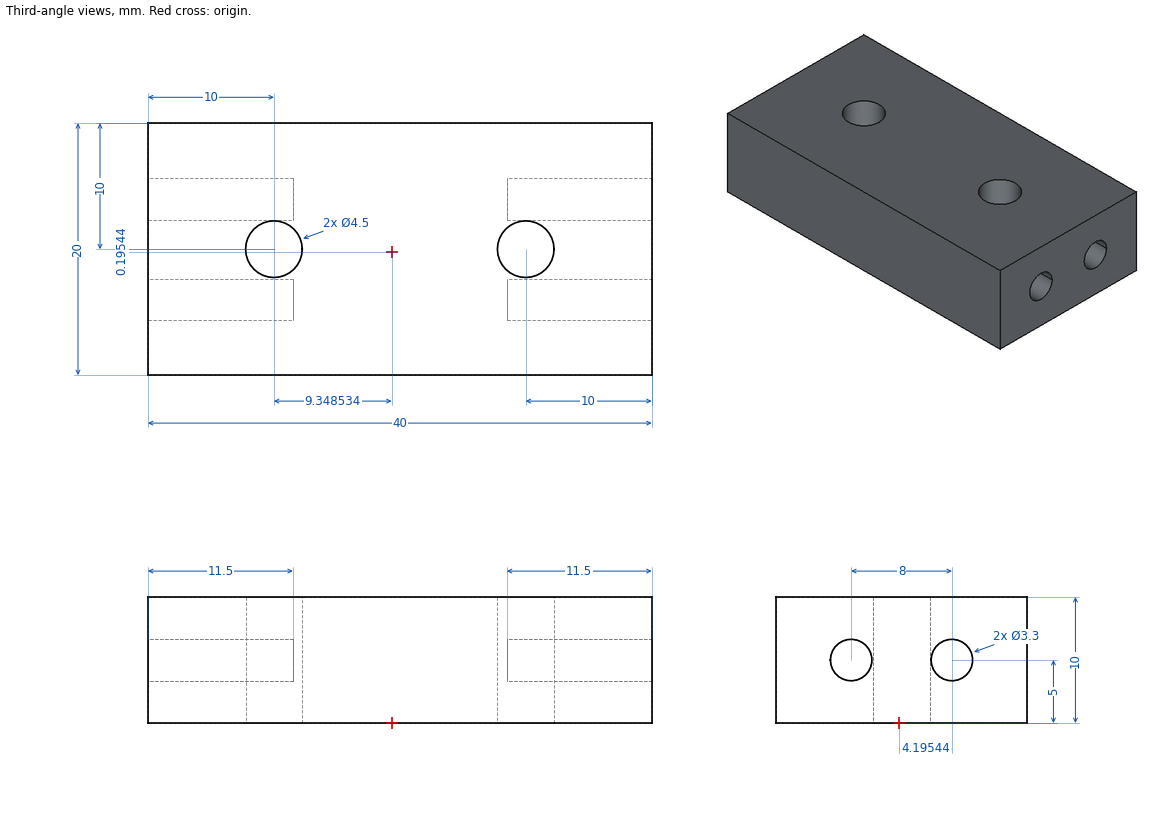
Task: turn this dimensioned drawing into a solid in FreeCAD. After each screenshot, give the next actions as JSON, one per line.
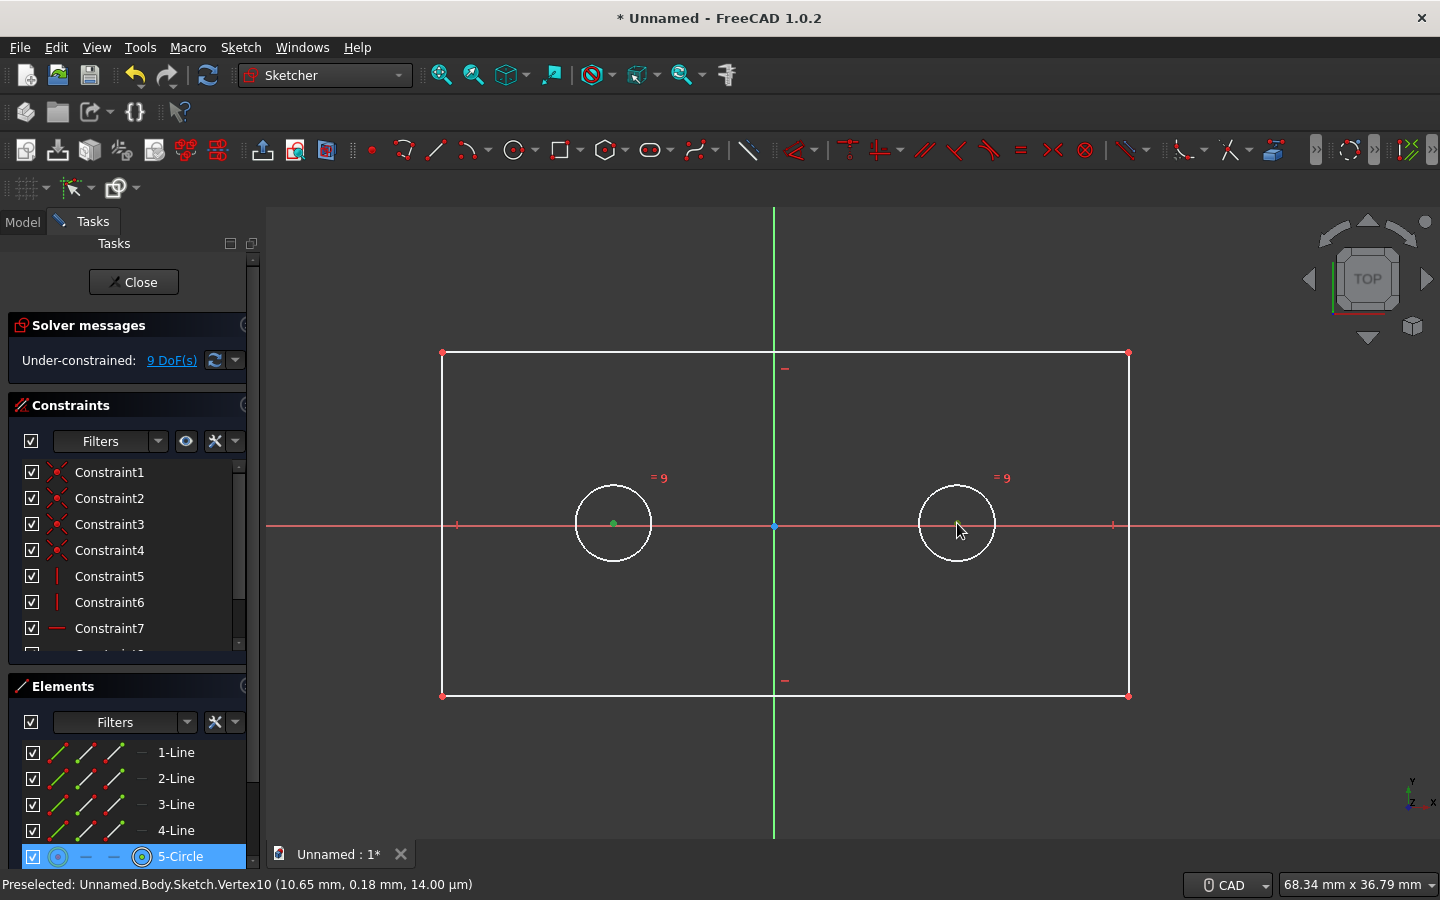
{"action": "key", "text": "h"}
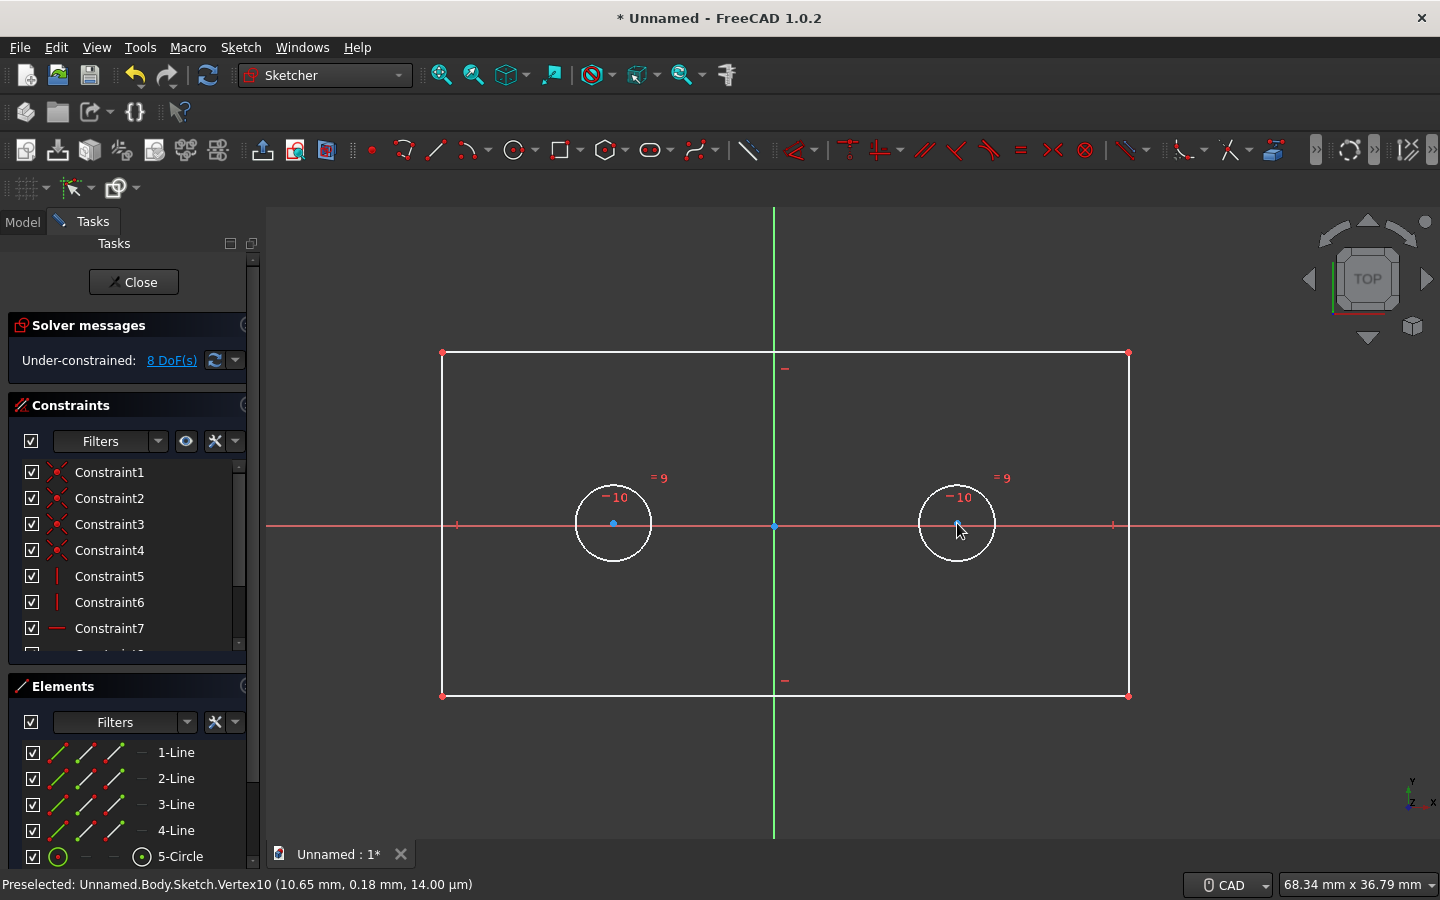
{"action": "key", "text": "d"}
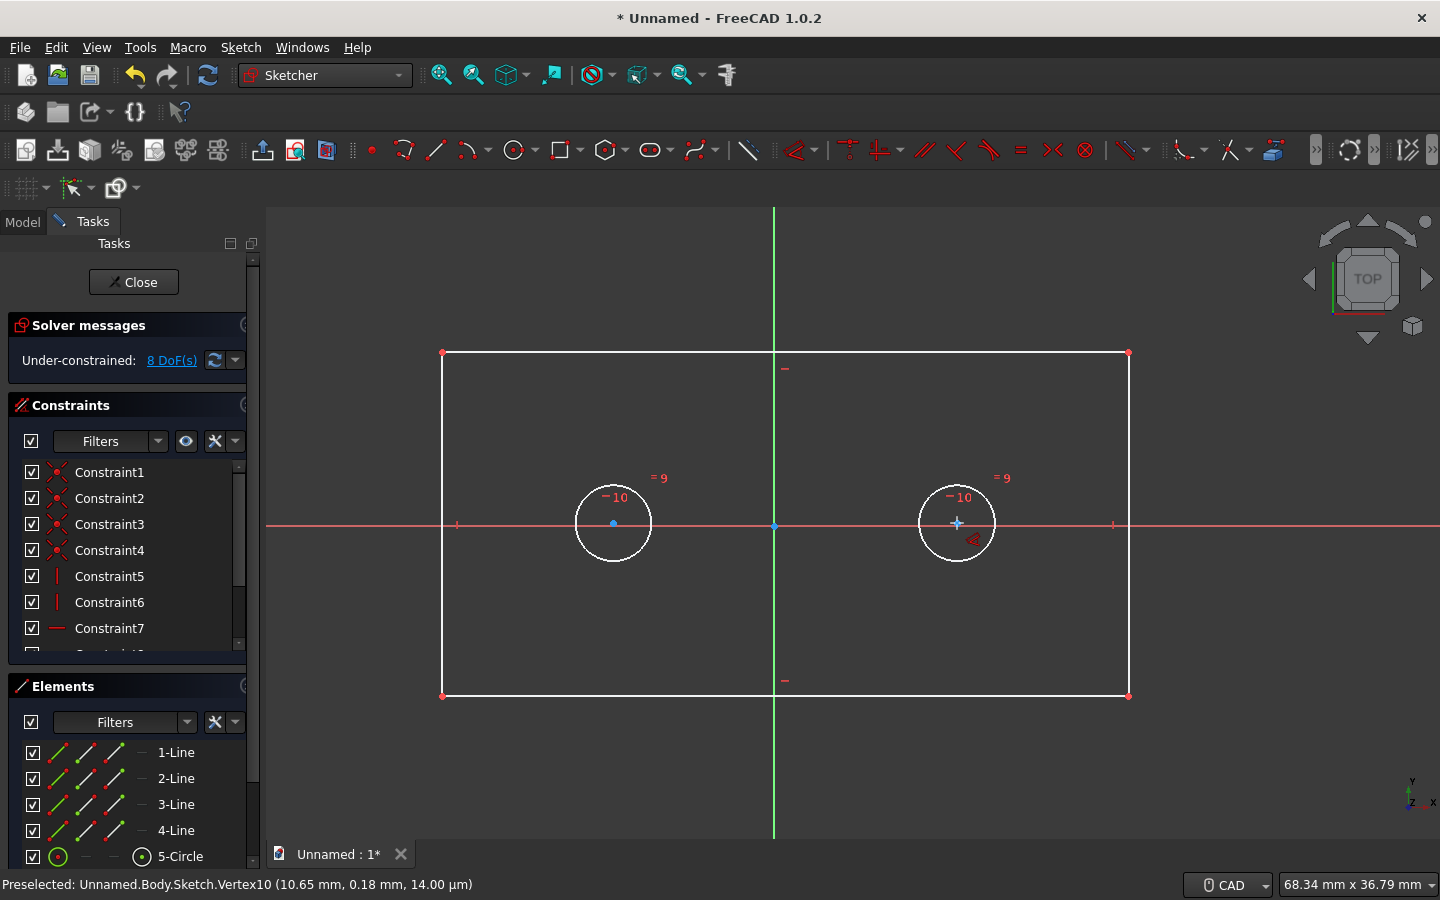
{"action": "left_click", "coordinate": [640, 496]}
{"action": "left_click", "coordinate": [662, 473]}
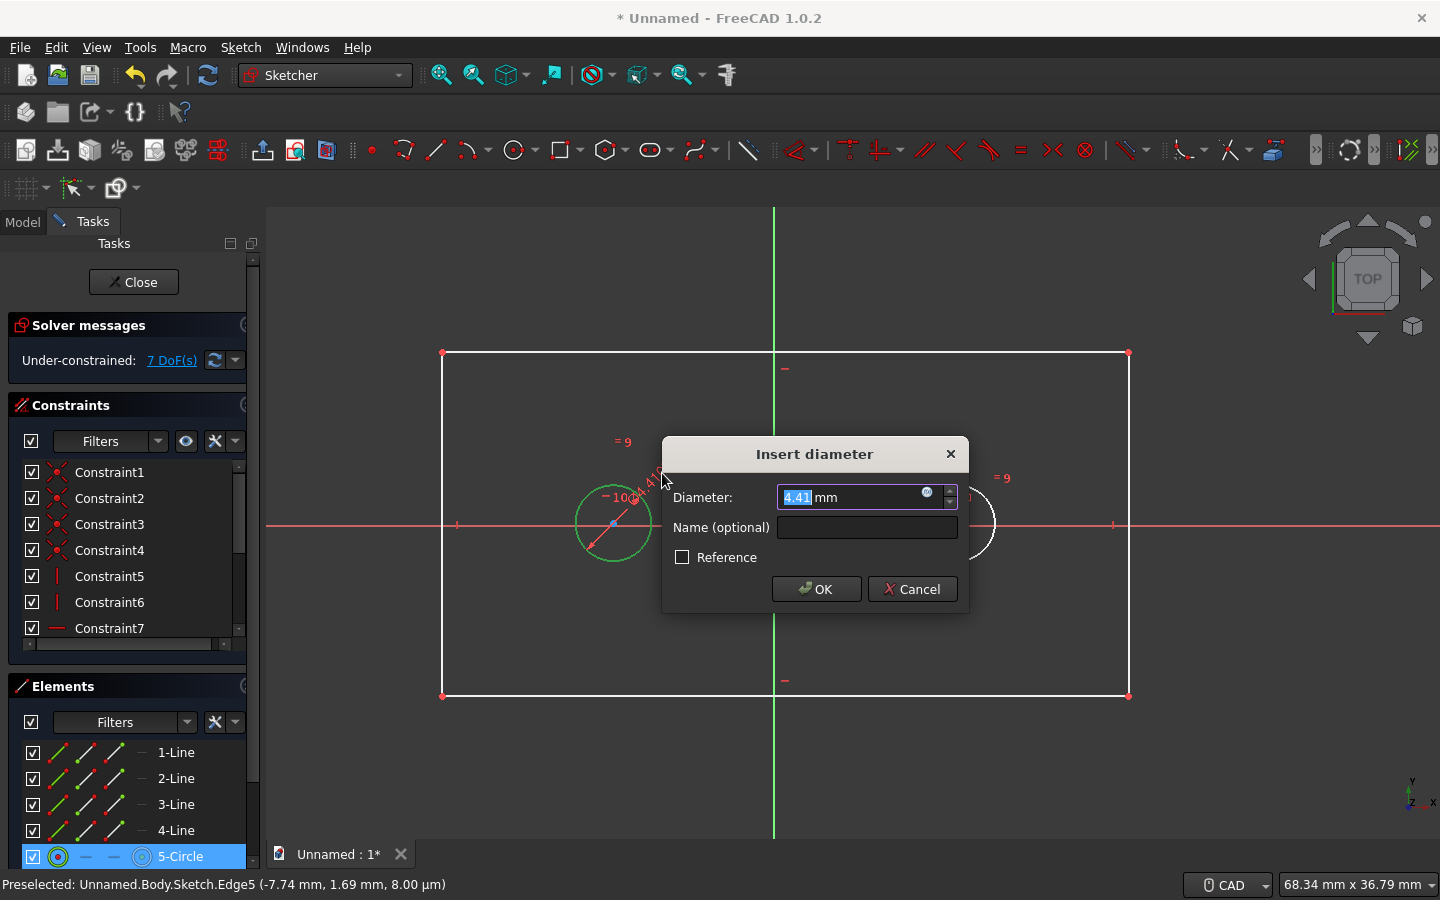
{"action": "type", "text": "4.5"}
{"action": "key", "text": "Return"}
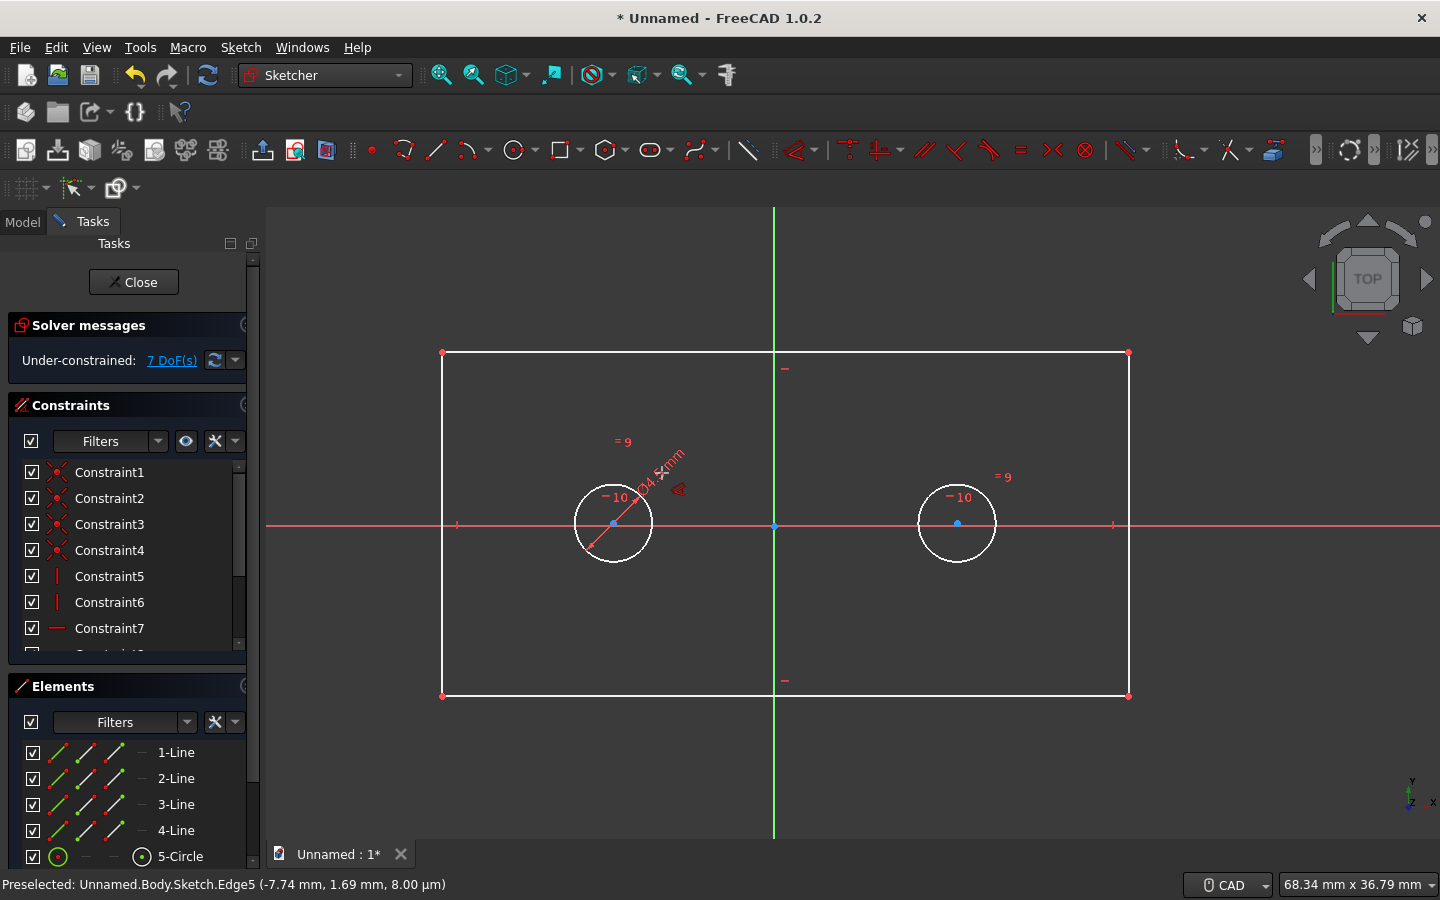
{"action": "left_click", "coordinate": [442, 456]}
{"action": "left_click", "coordinate": [408, 445]}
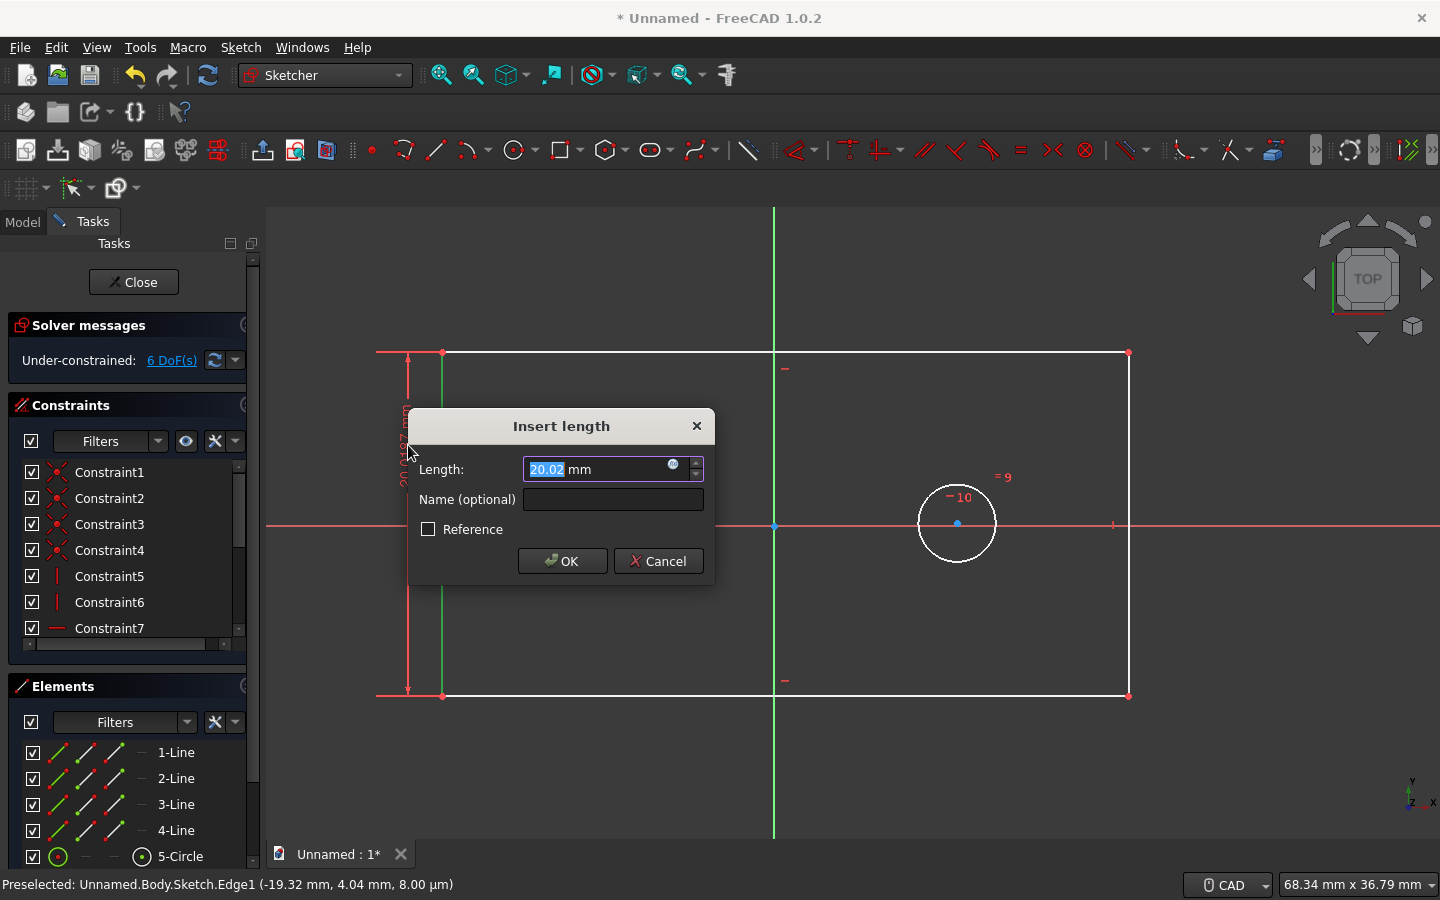
{"action": "type", "text": "20"}
{"action": "key", "text": "Return"}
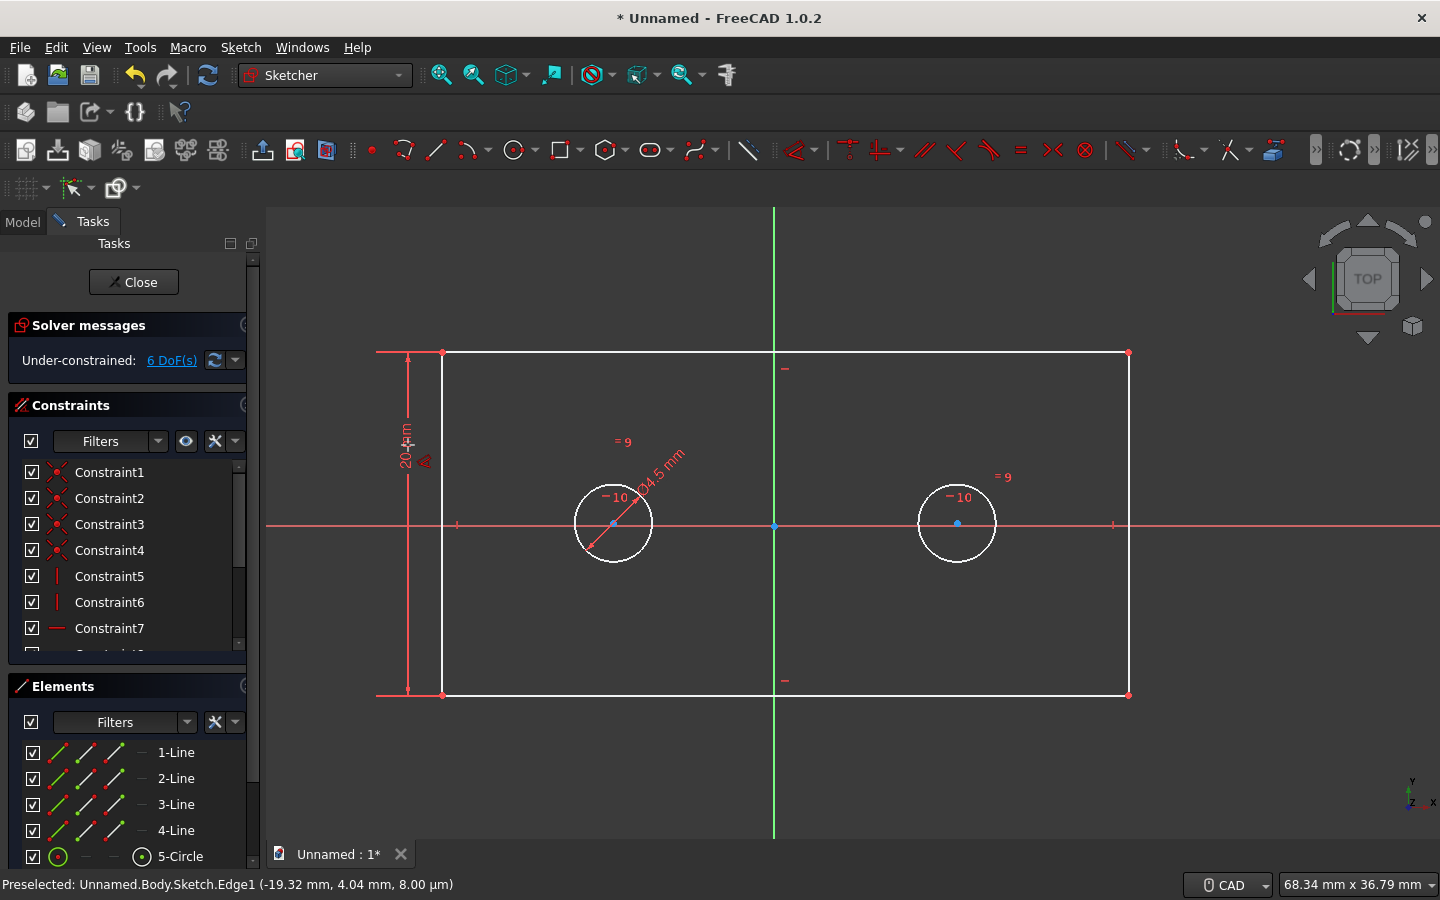
{"action": "left_click", "coordinate": [648, 696]}
{"action": "left_click", "coordinate": [628, 730]}